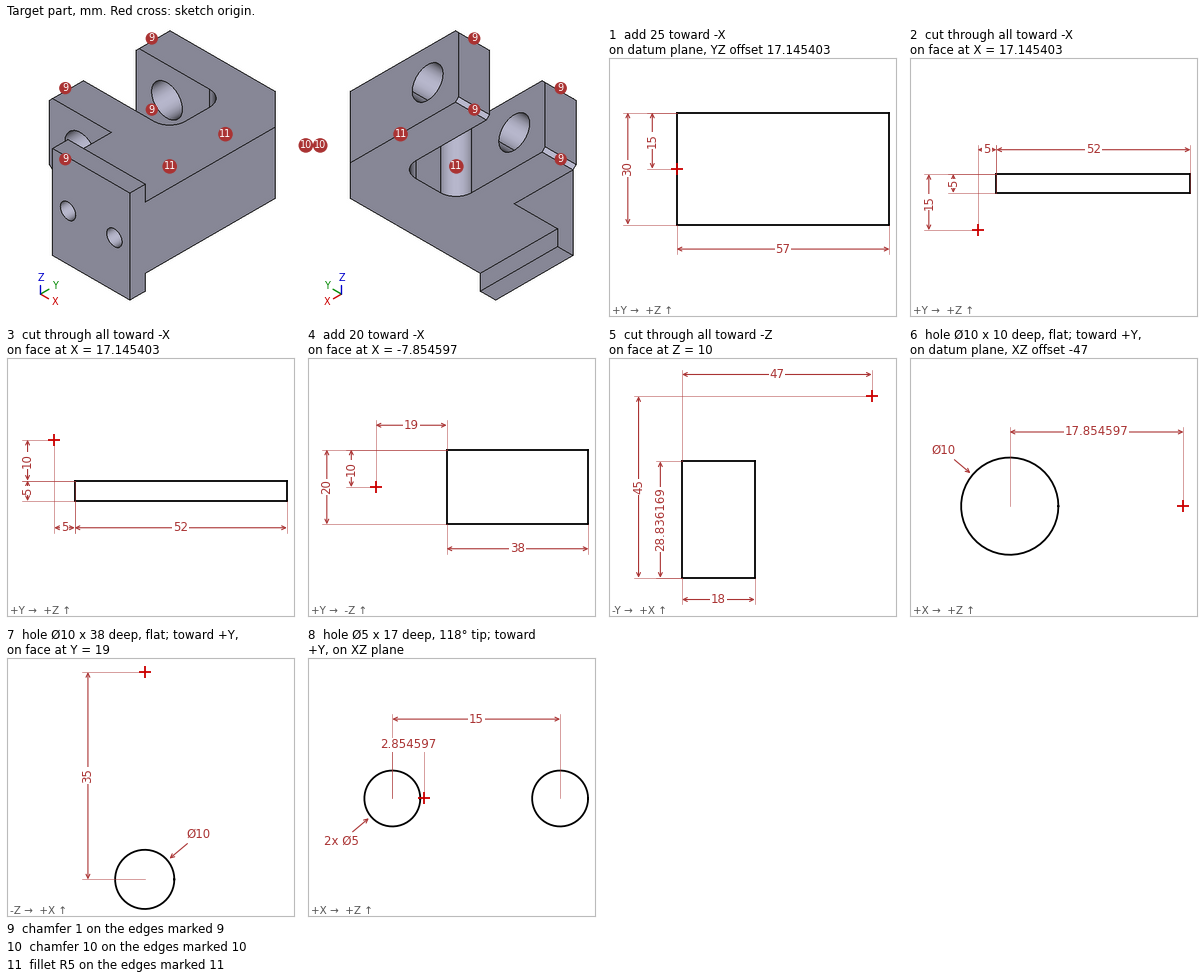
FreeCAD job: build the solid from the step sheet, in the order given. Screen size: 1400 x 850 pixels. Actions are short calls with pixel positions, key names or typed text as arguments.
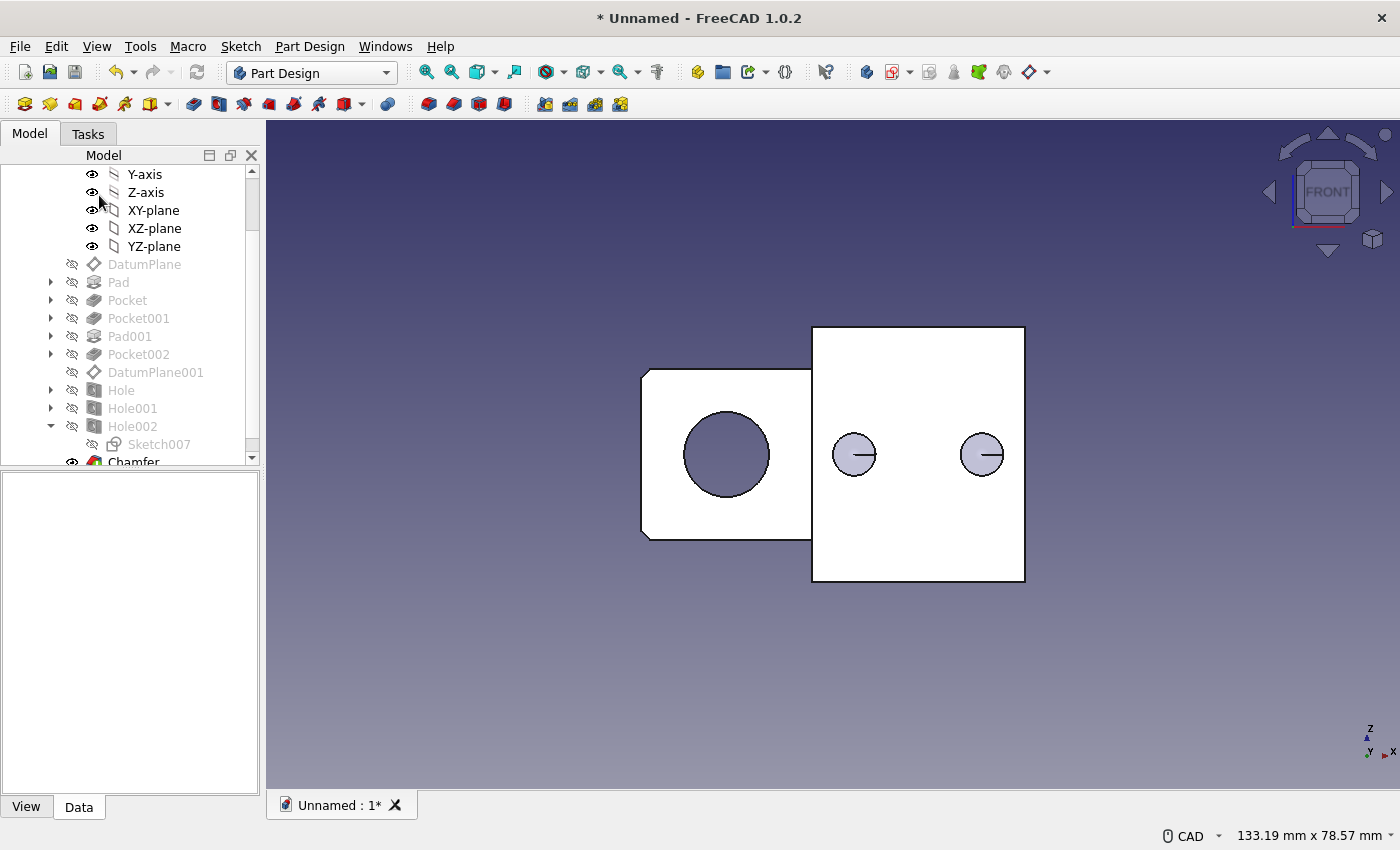
key(3)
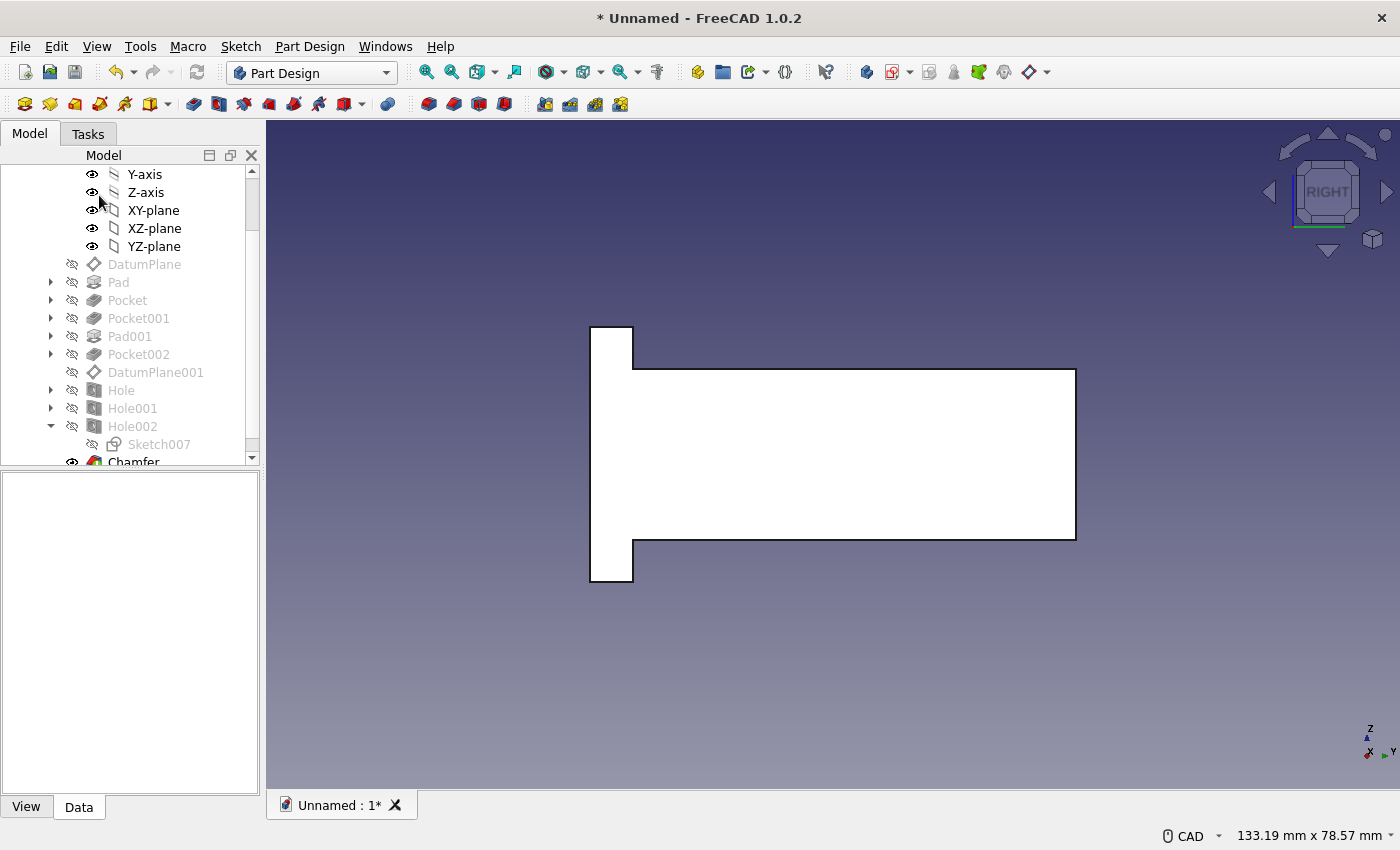
click(427, 72)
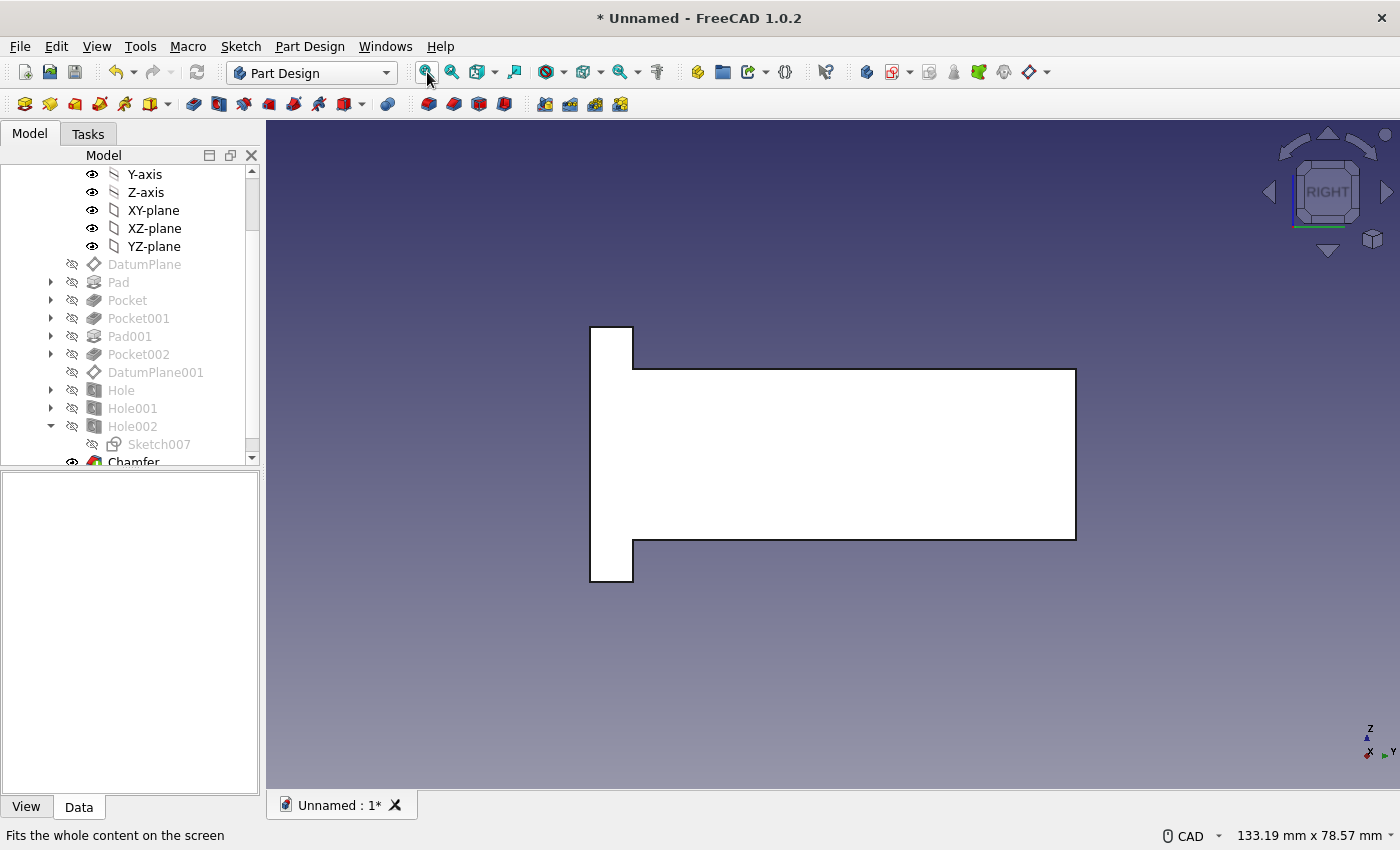
click(1076, 453)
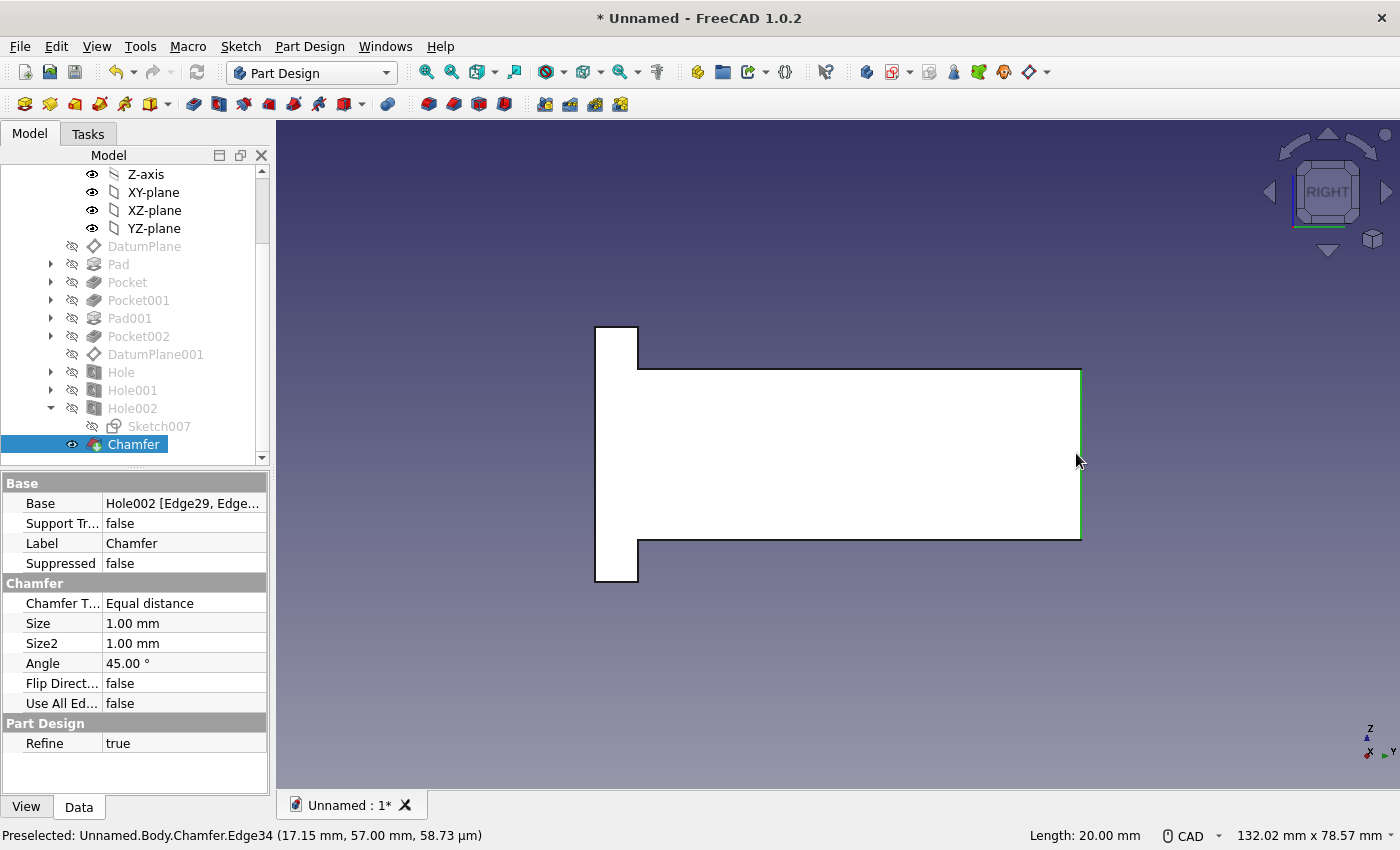
click(454, 104)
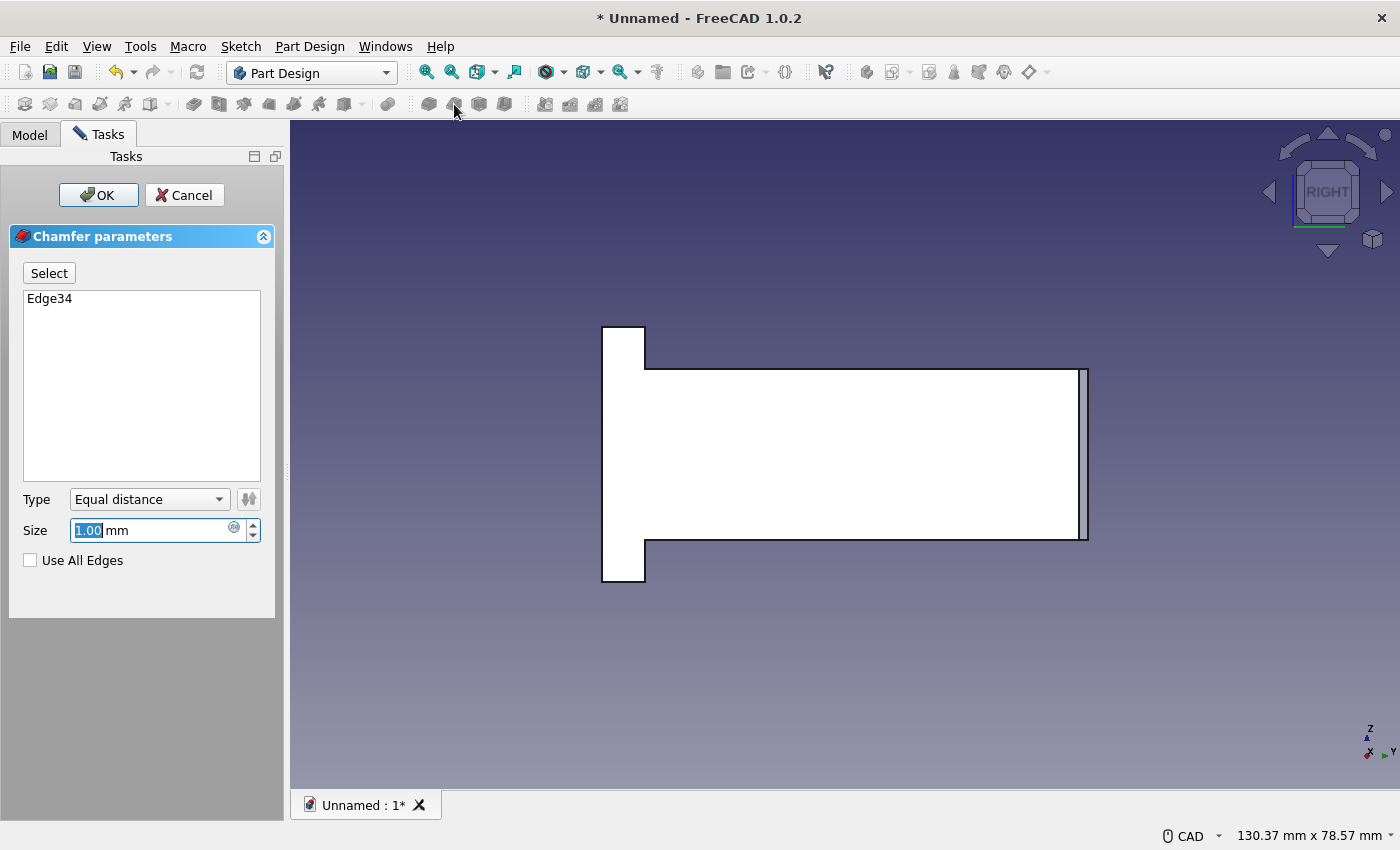
text(10)
key(Tab)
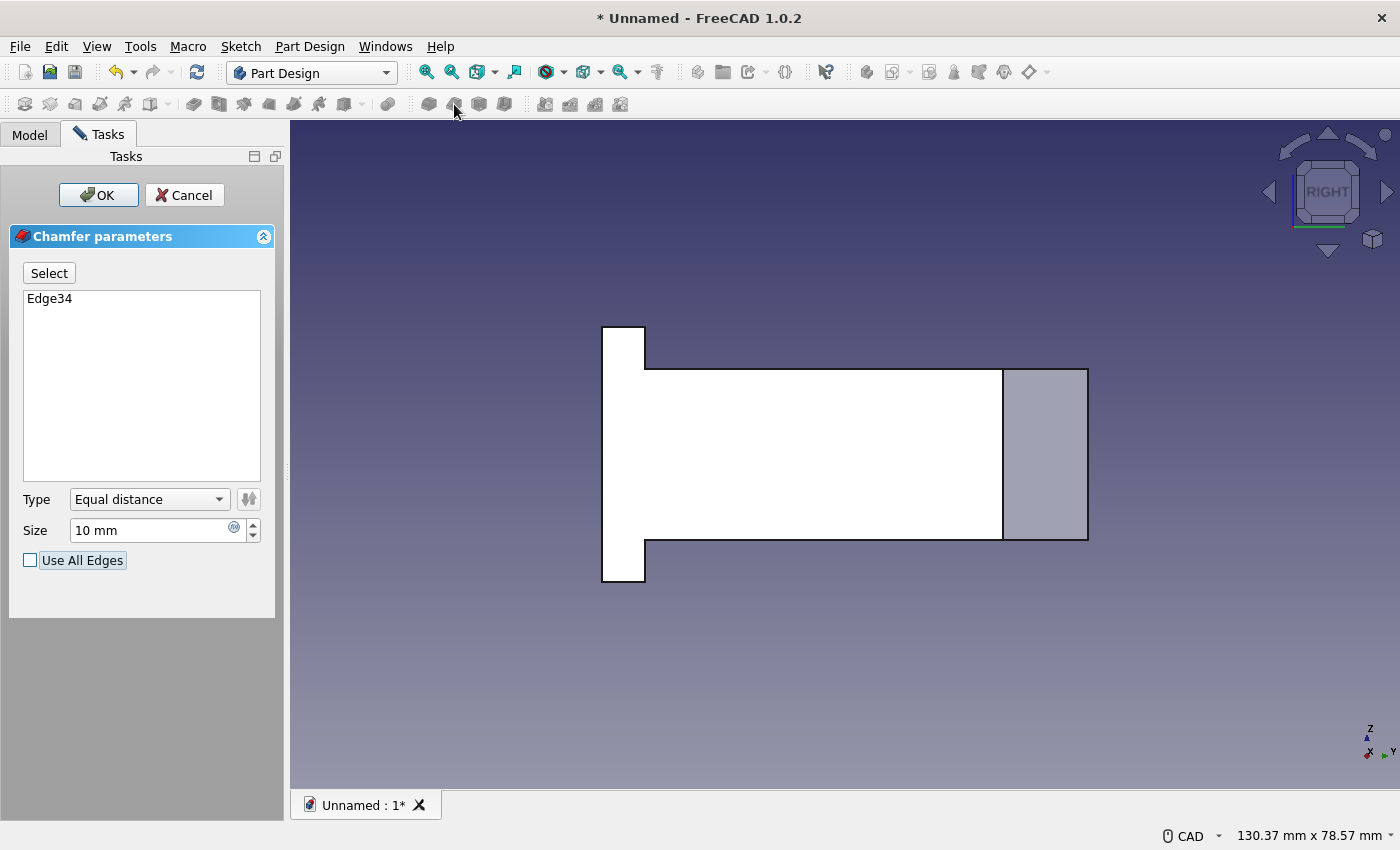
click(99, 195)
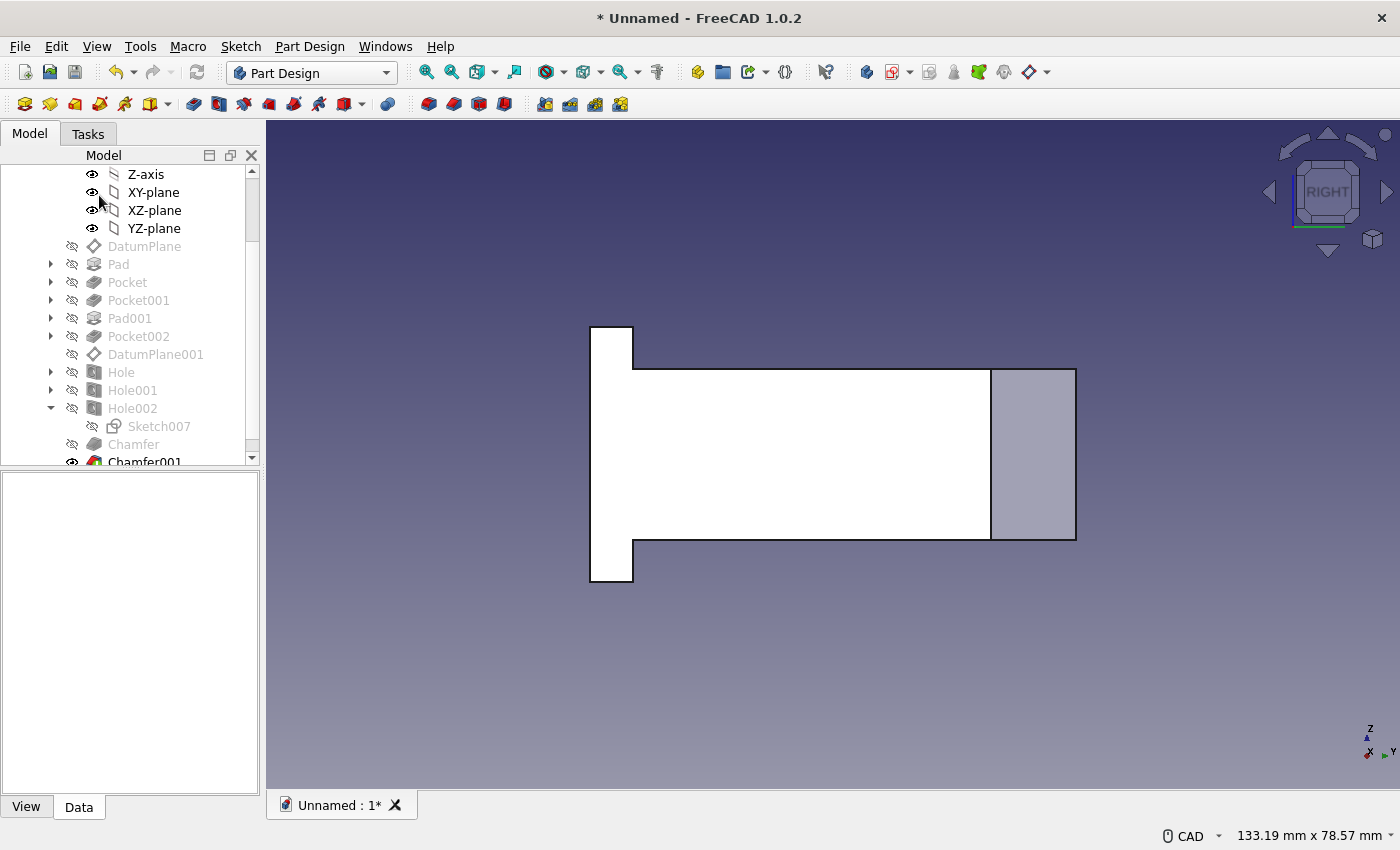
key(v)
key(f)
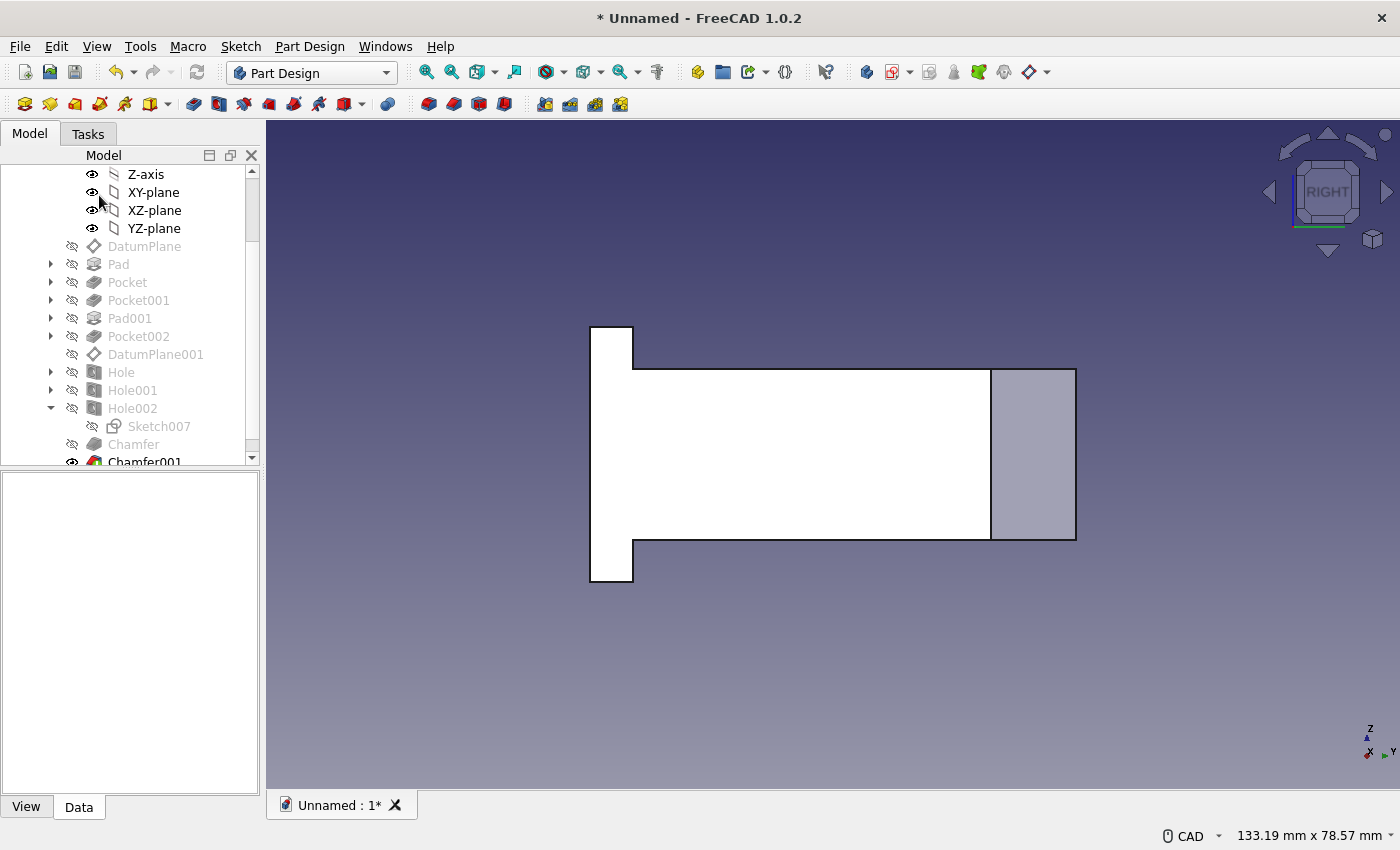
key(0)